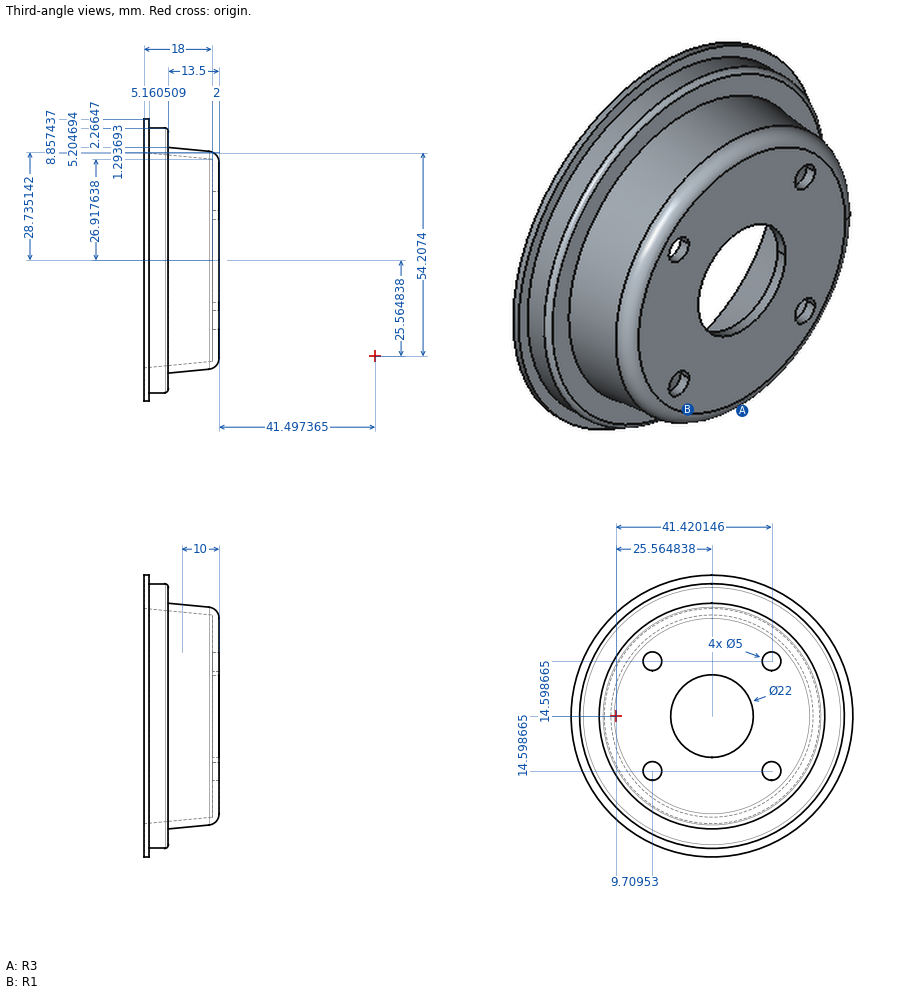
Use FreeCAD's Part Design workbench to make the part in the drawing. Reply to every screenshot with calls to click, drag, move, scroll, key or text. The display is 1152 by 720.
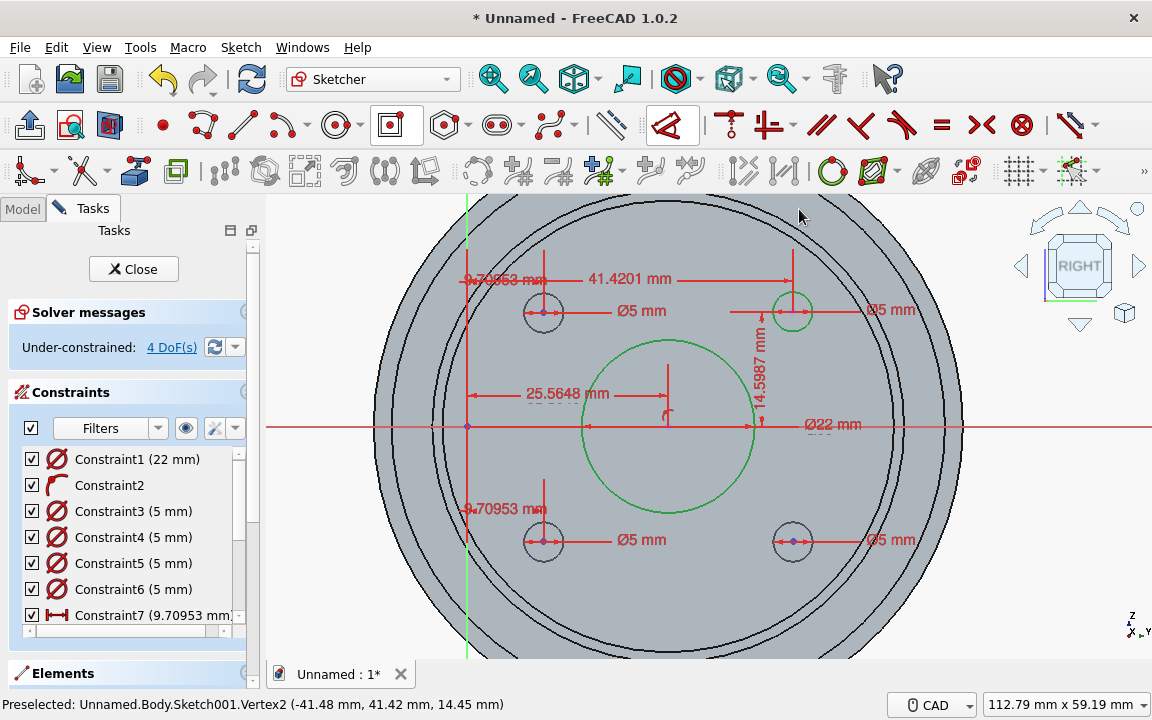
click(793, 542)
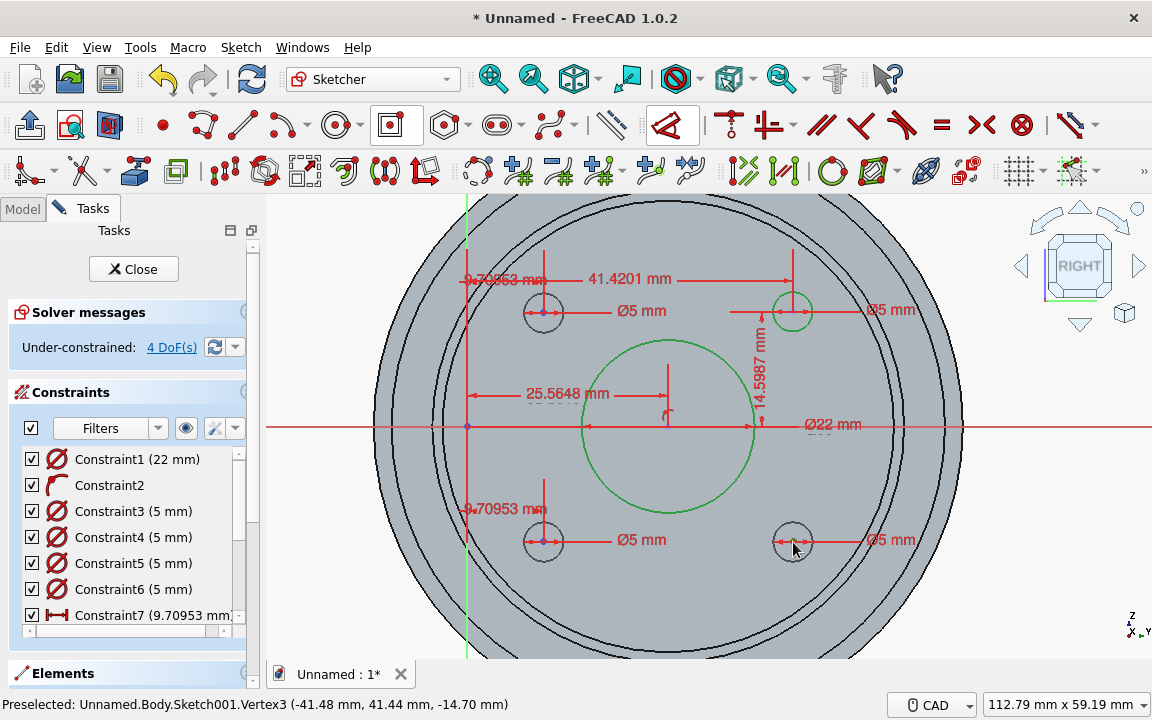
key(l)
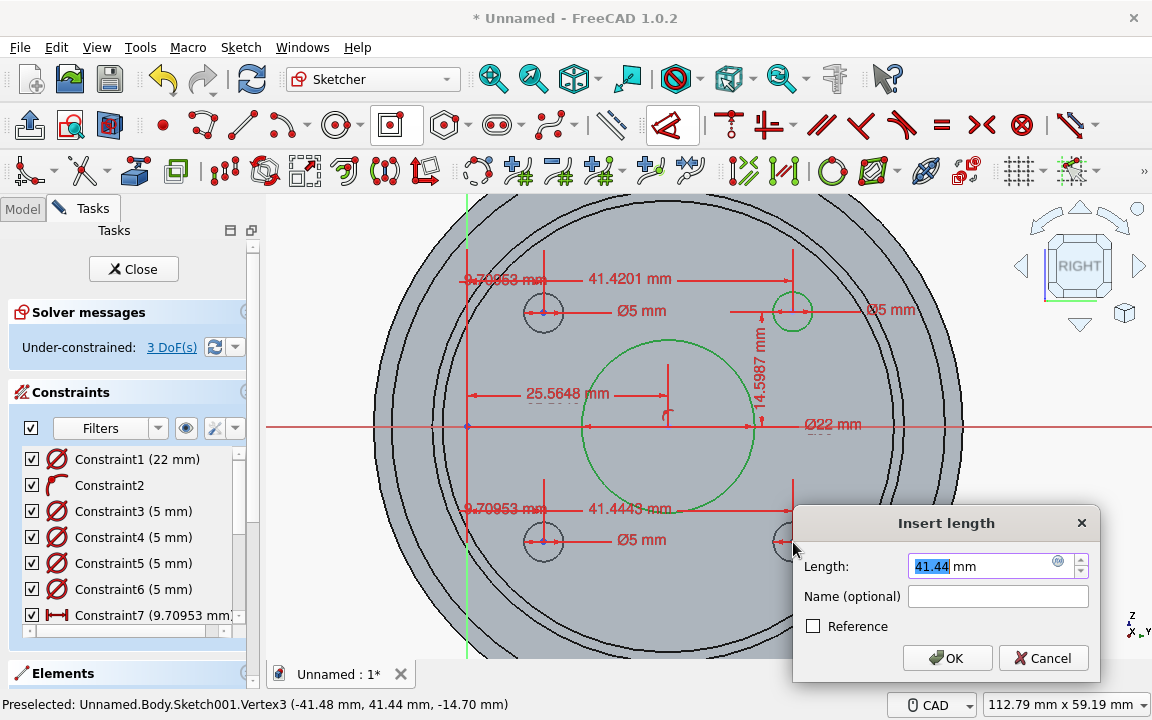
text(41.420146)
key(Return)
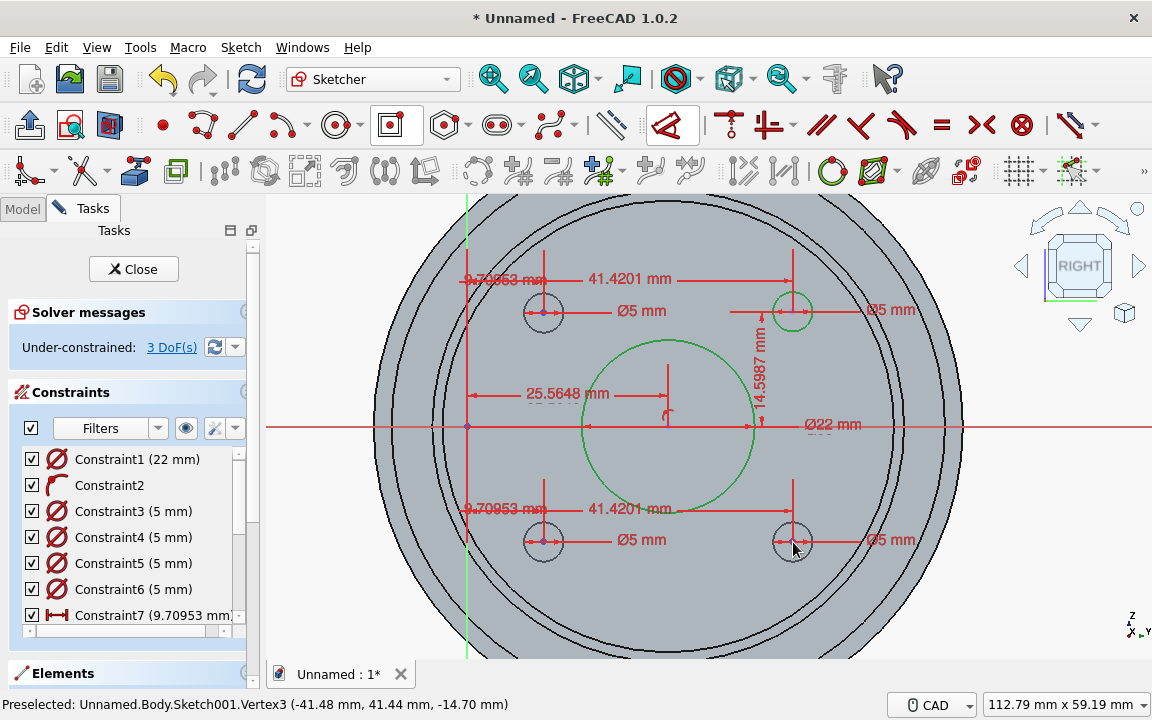
click(793, 542)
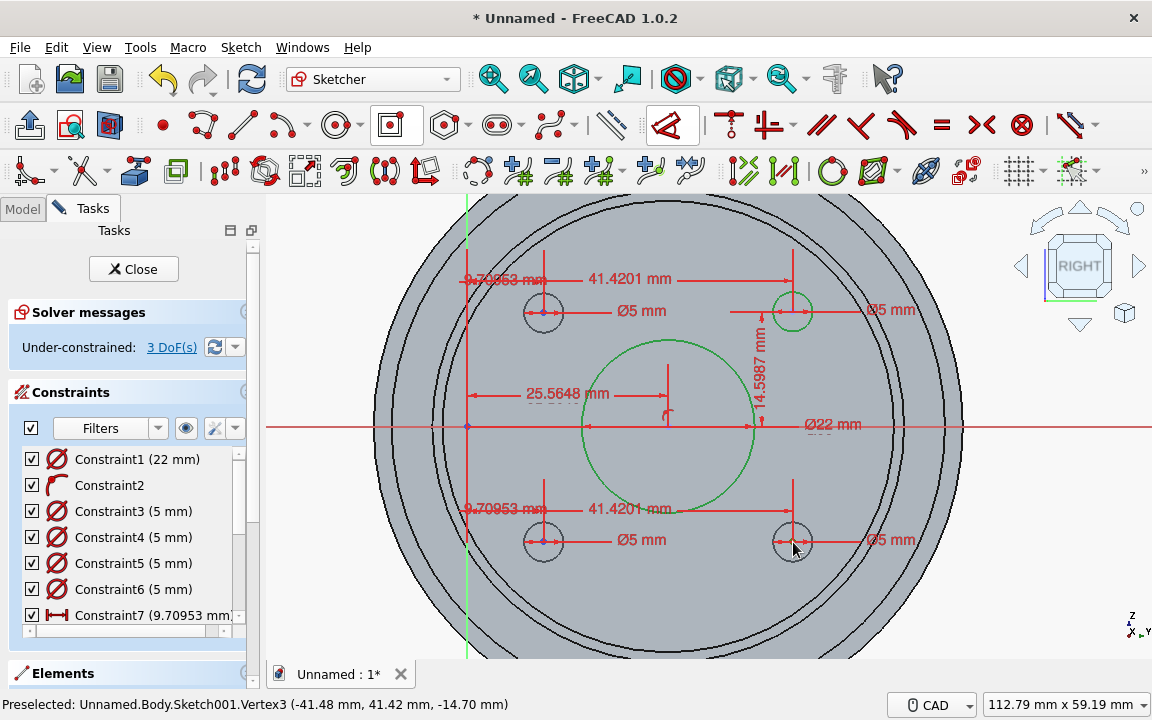
key(i)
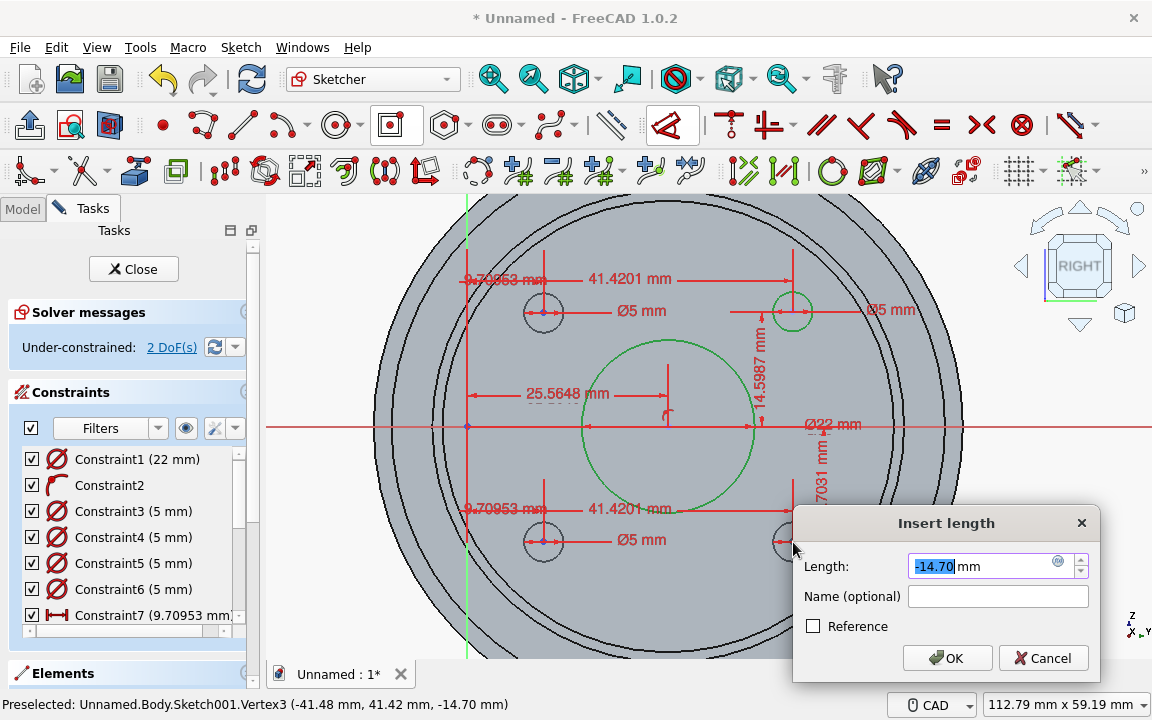
text(-14.598665)
key(Return)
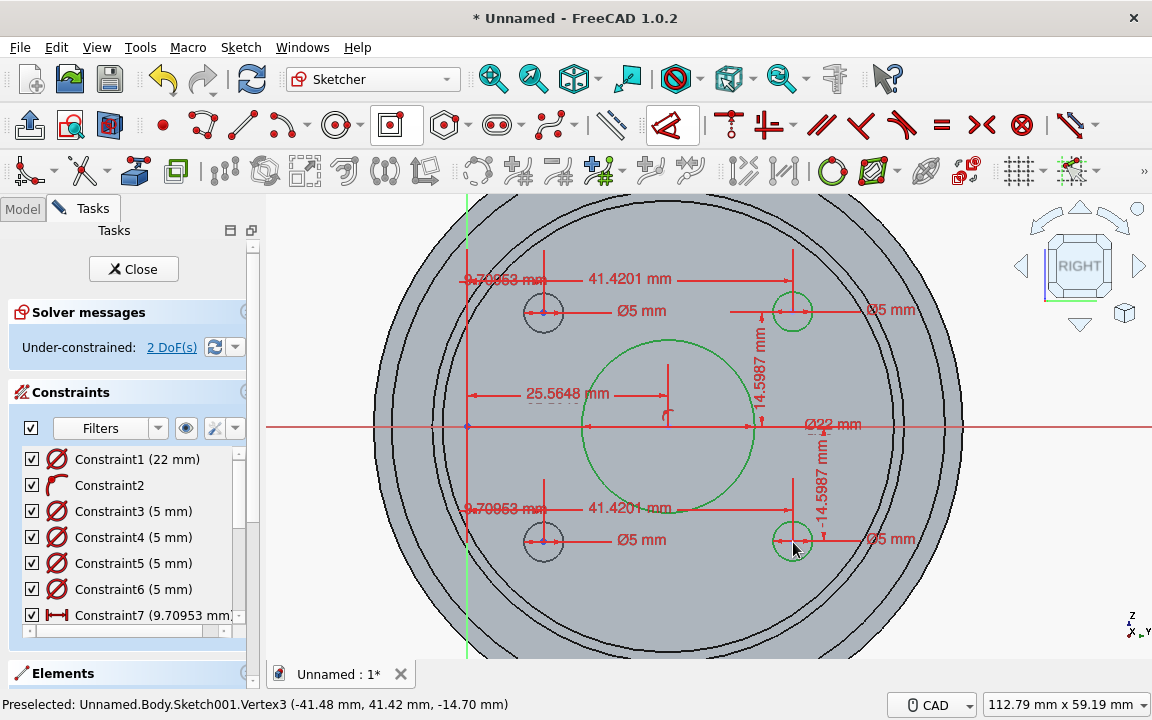
click(544, 542)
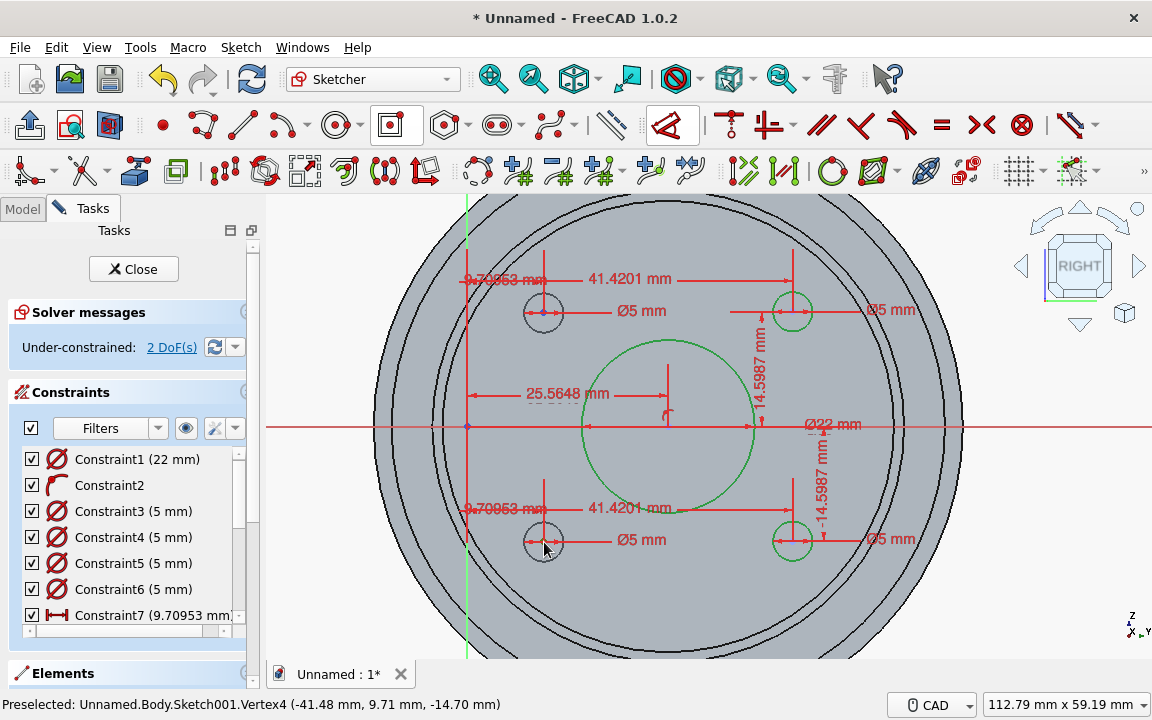
click(694, 126)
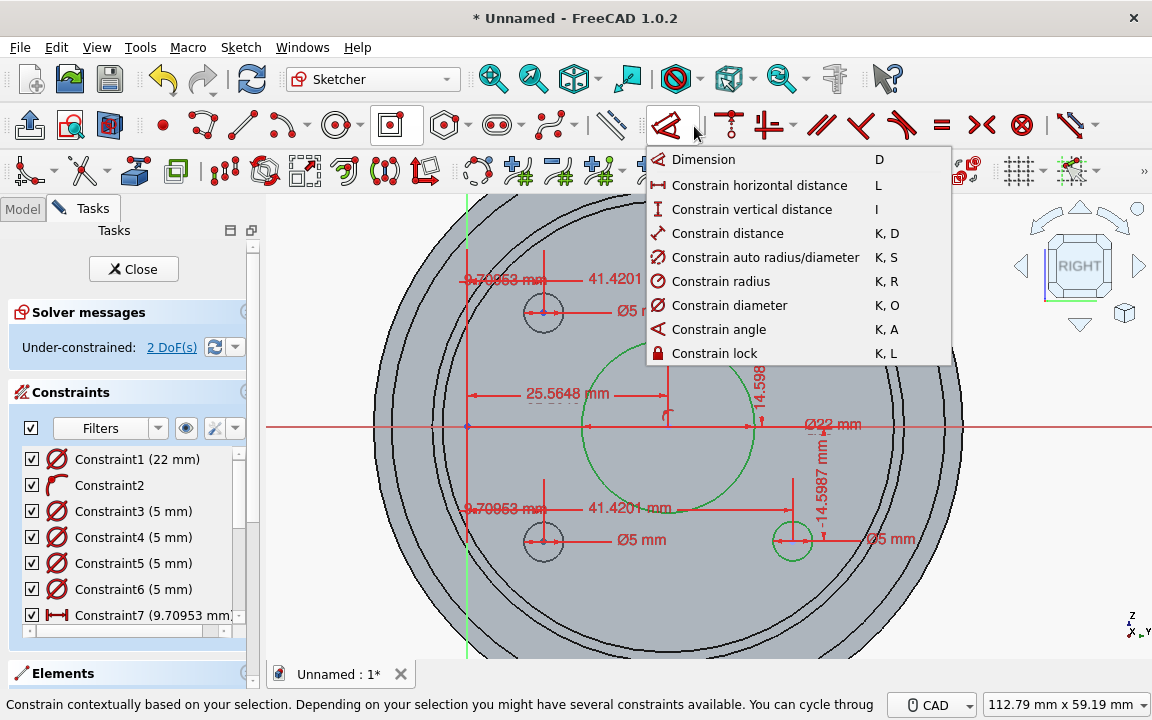
click(799, 209)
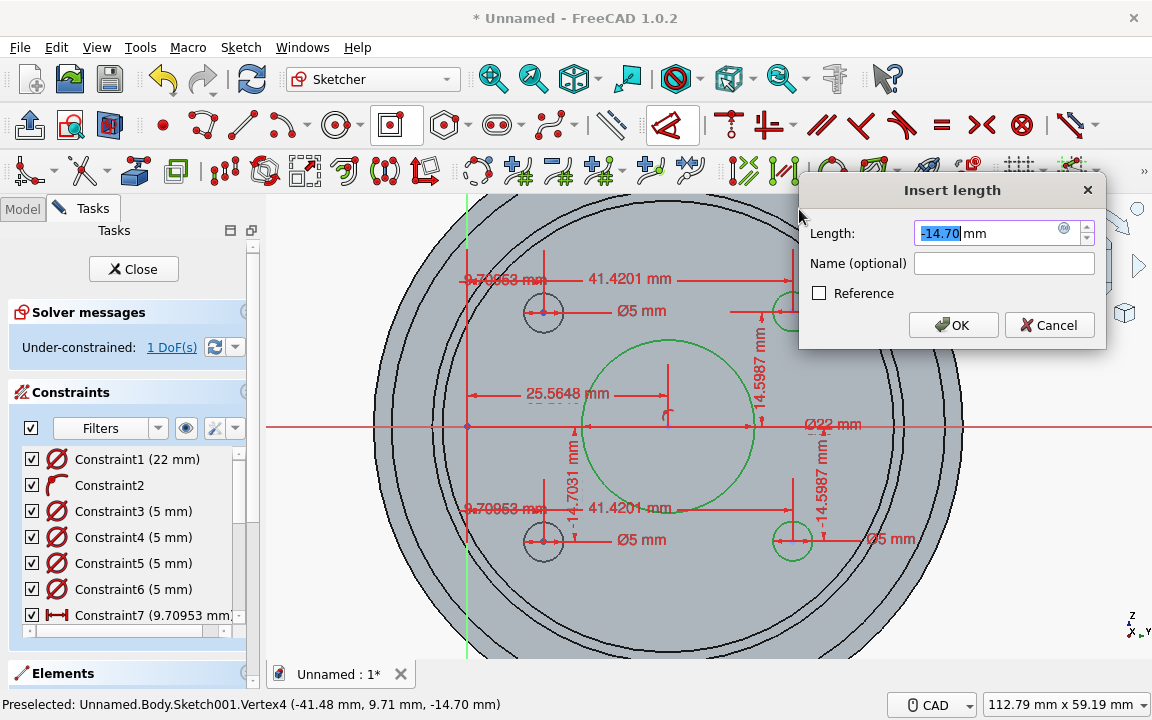
text(-14.598665)
key(Return)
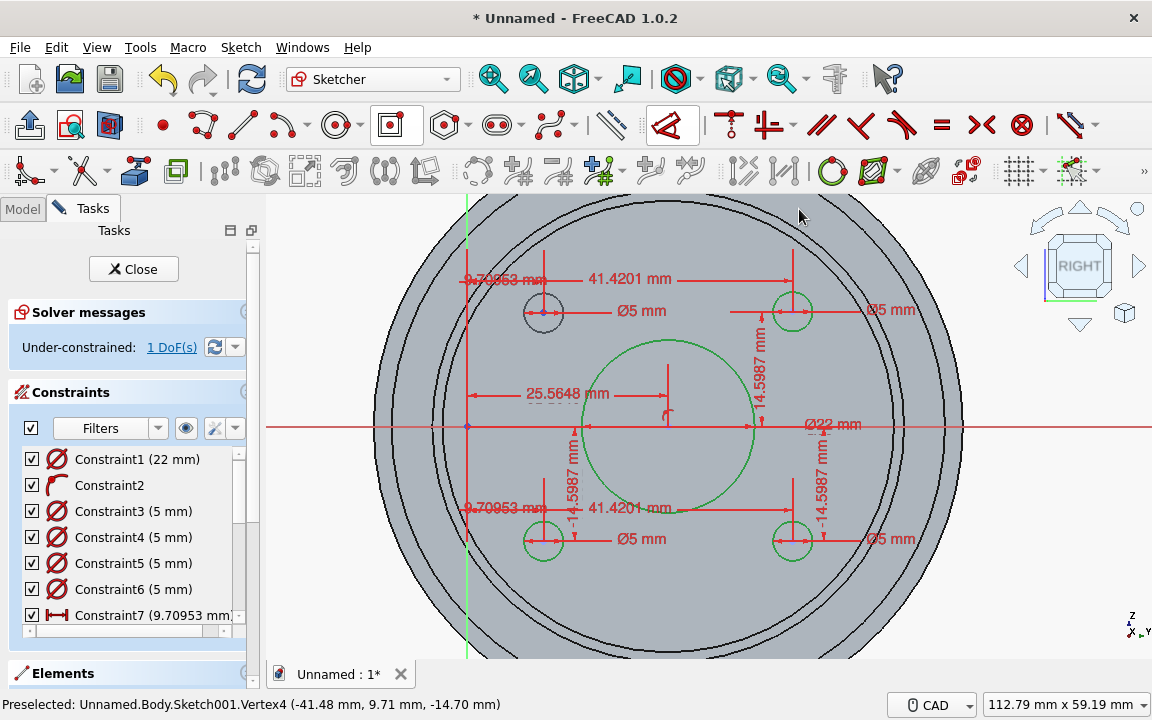
click(544, 313)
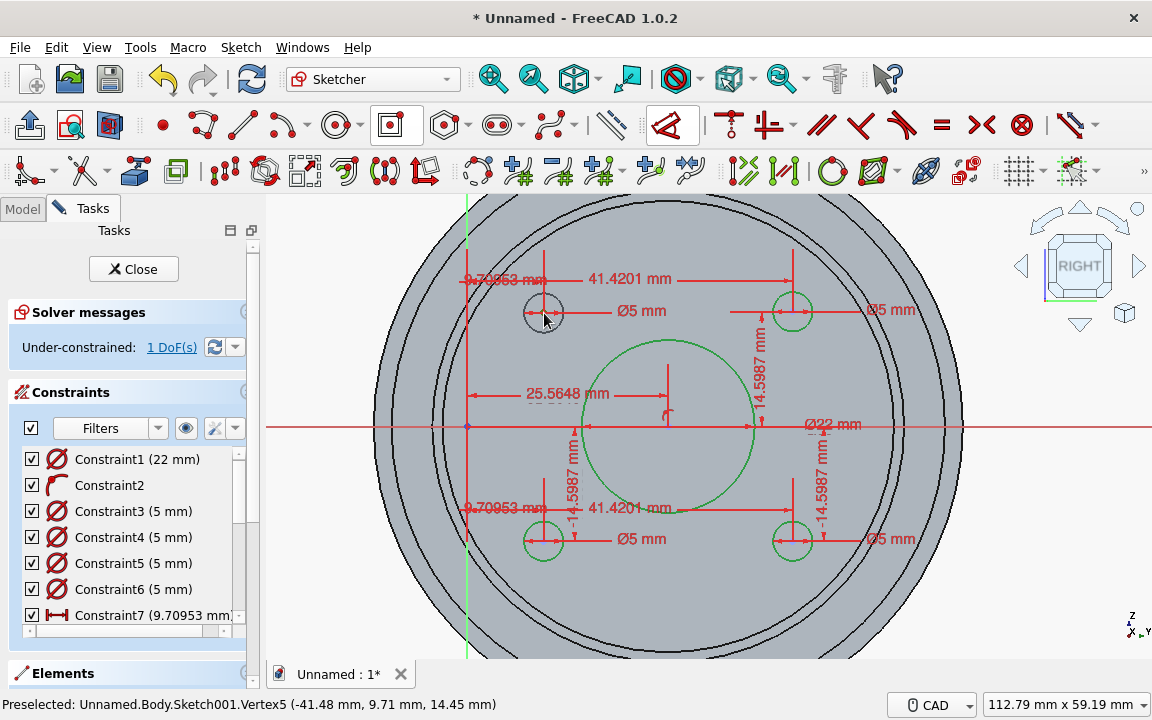
key(i)